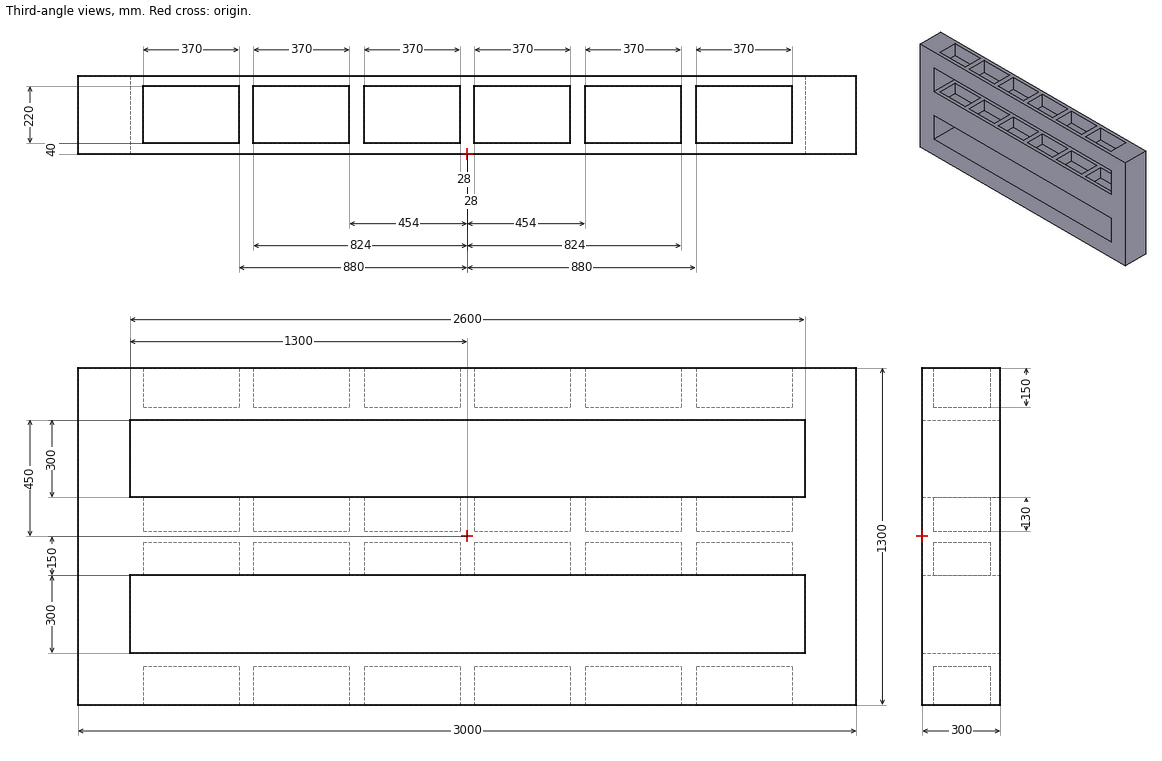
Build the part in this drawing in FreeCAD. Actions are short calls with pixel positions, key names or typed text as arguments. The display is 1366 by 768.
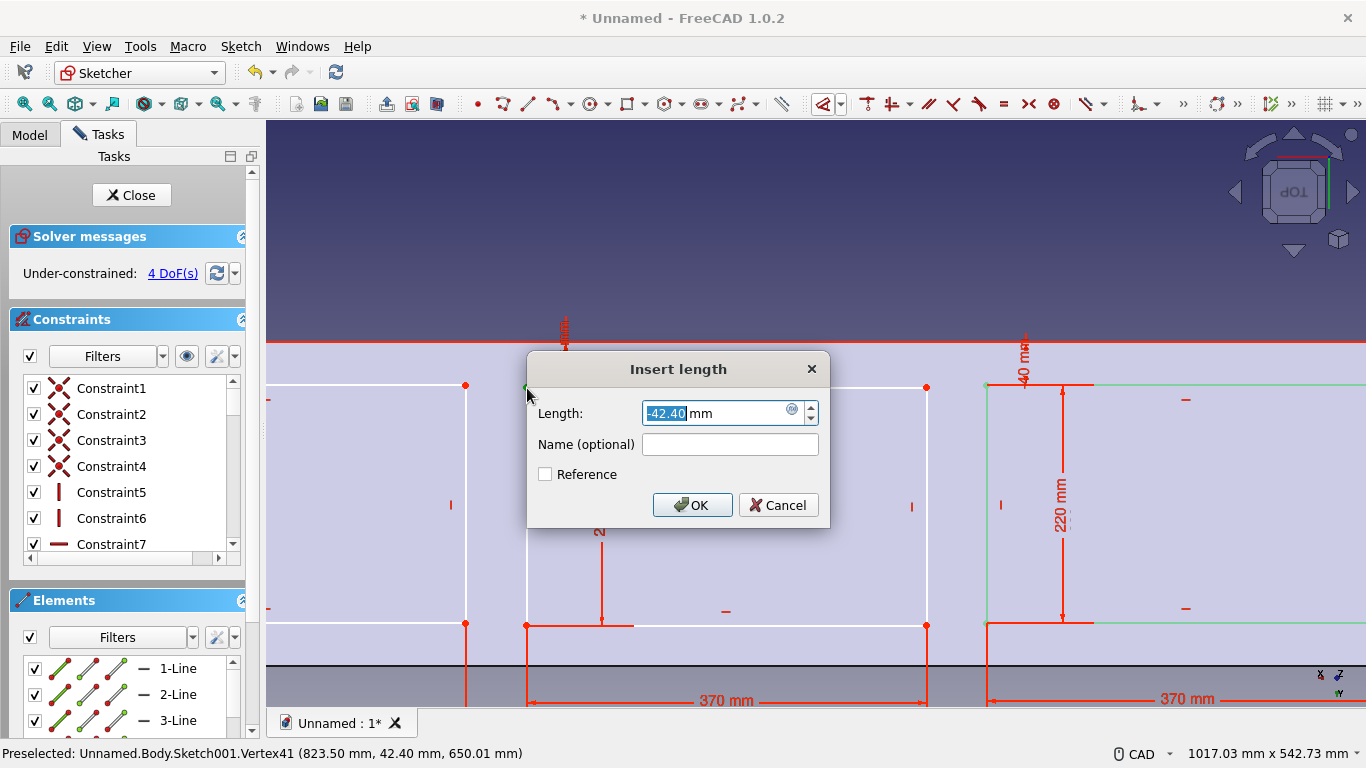
text(-40)
key(Return)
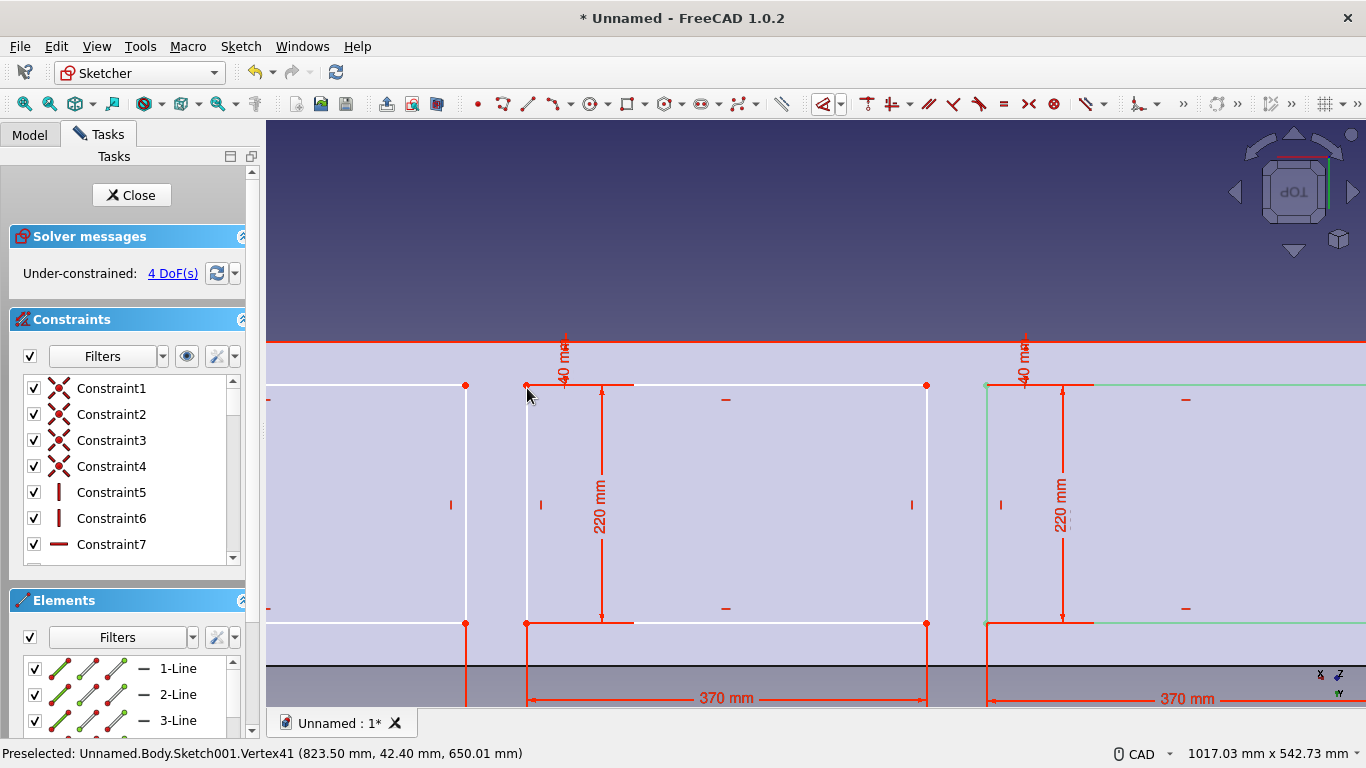
scroll(528, 391, down, 7)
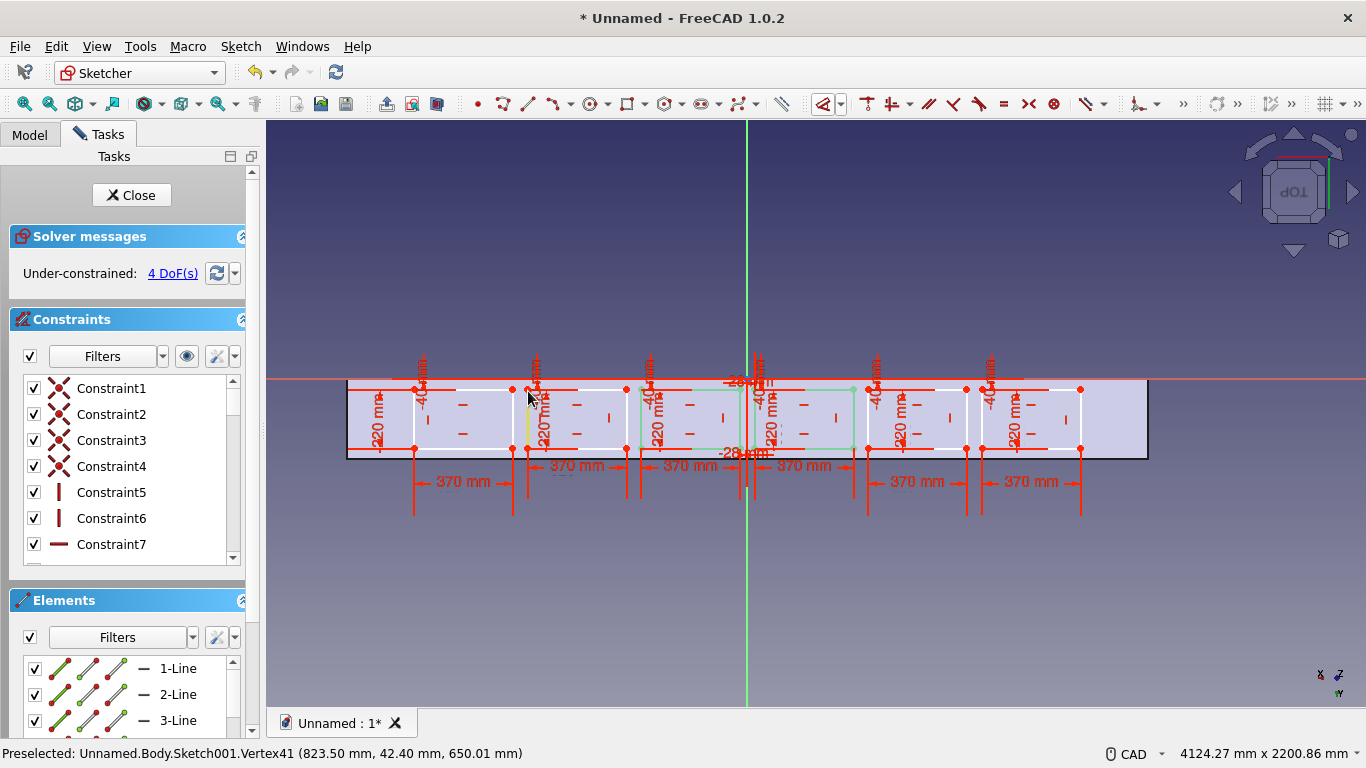
click(982, 390)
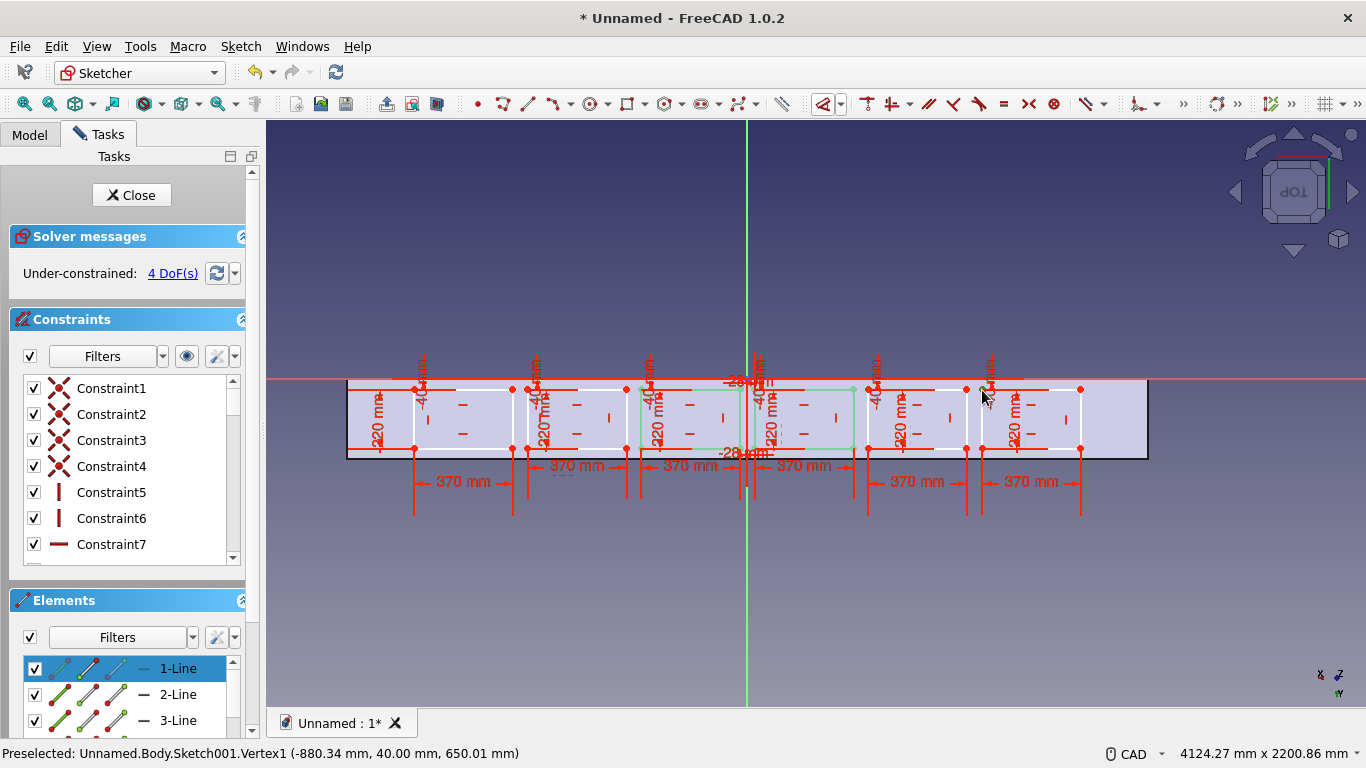
key(l)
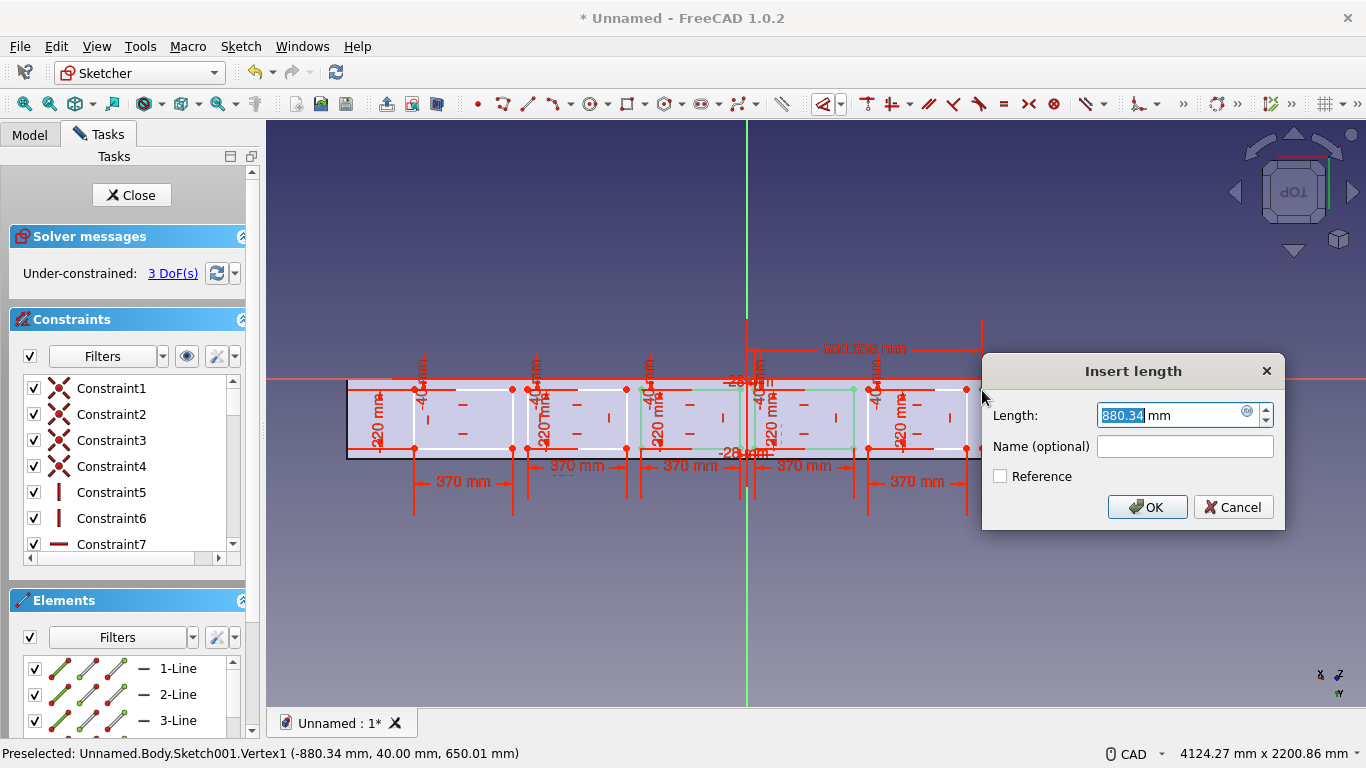
text(880)
key(Return)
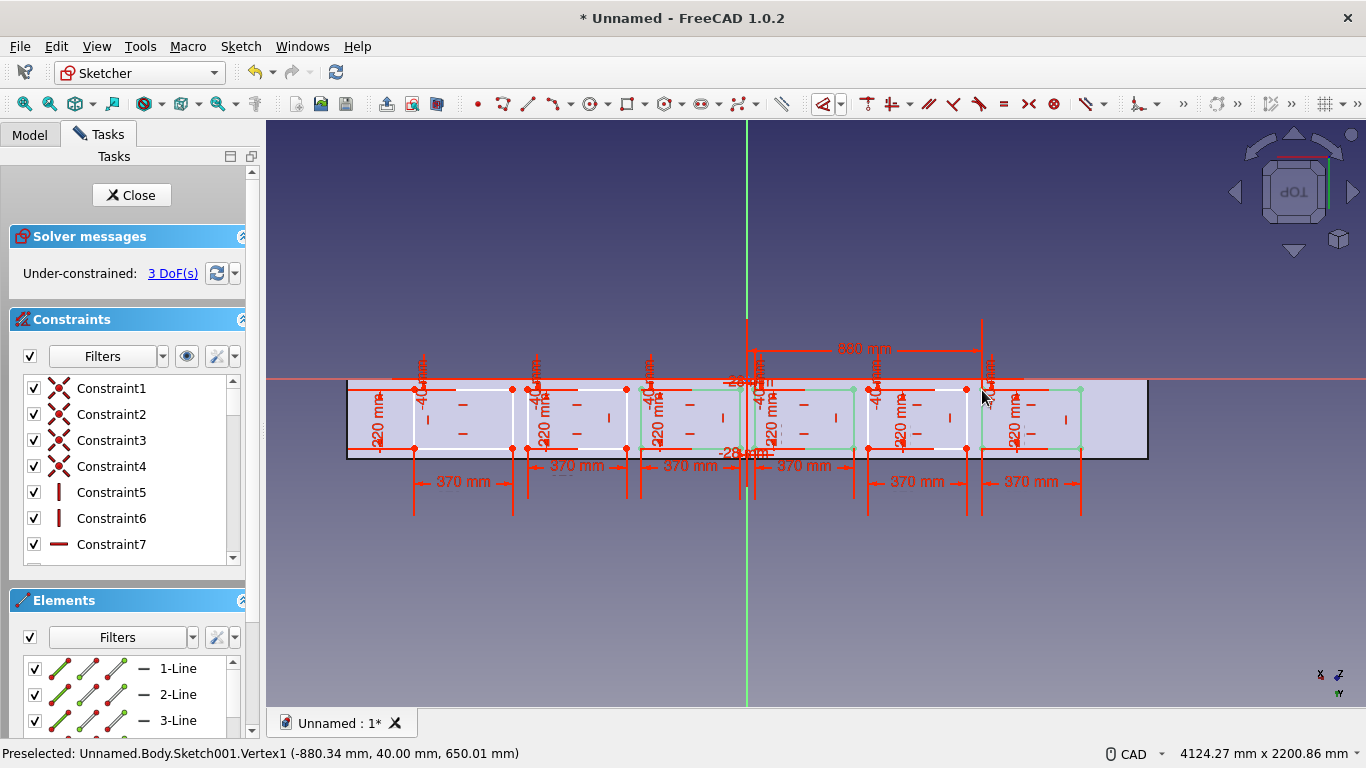
click(513, 449)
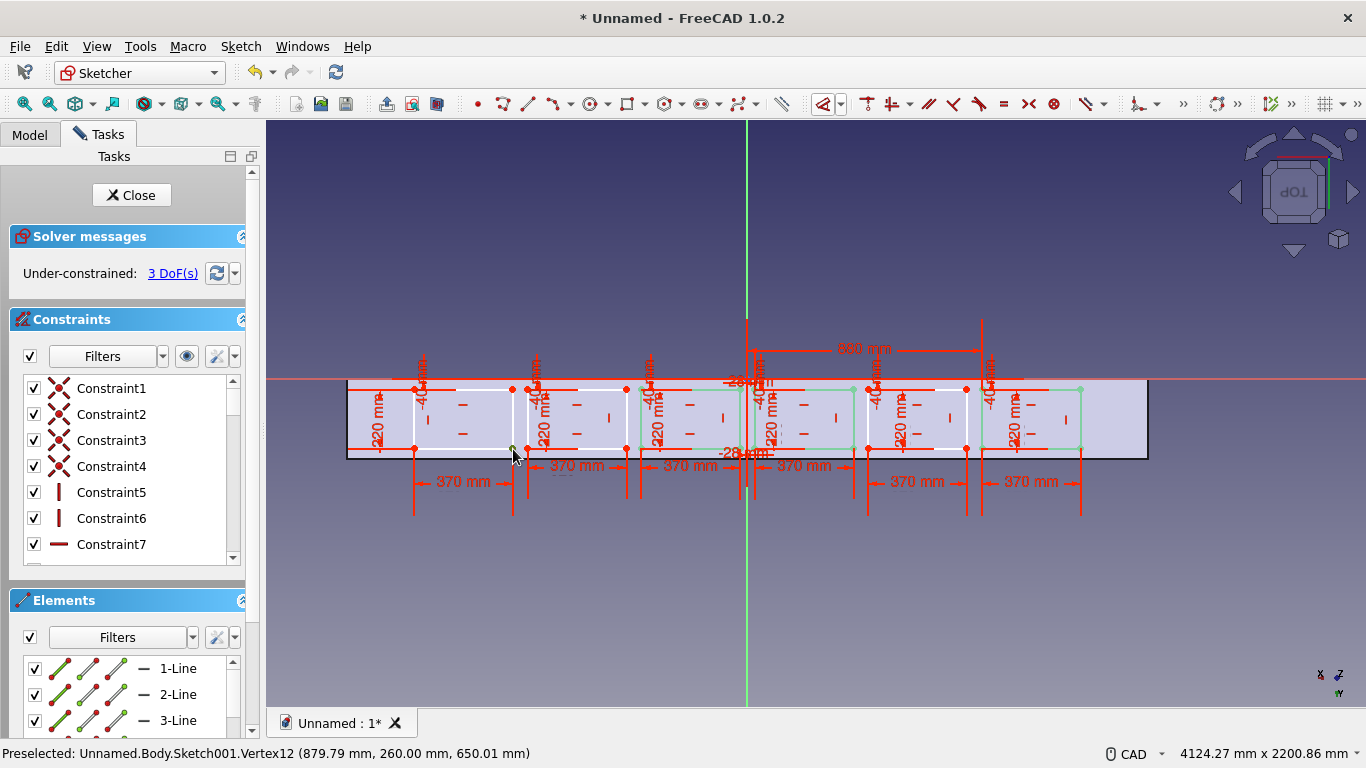
key(l)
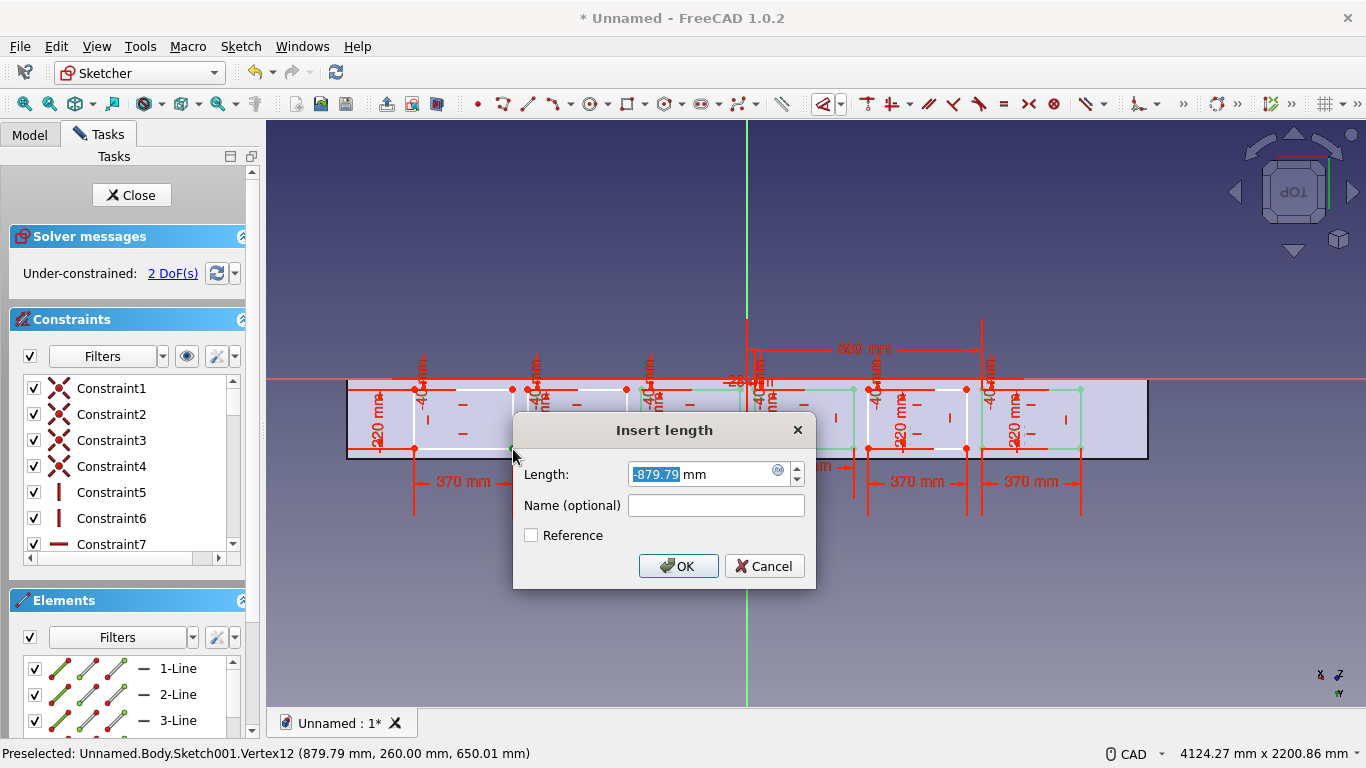
text(-880)
key(Return)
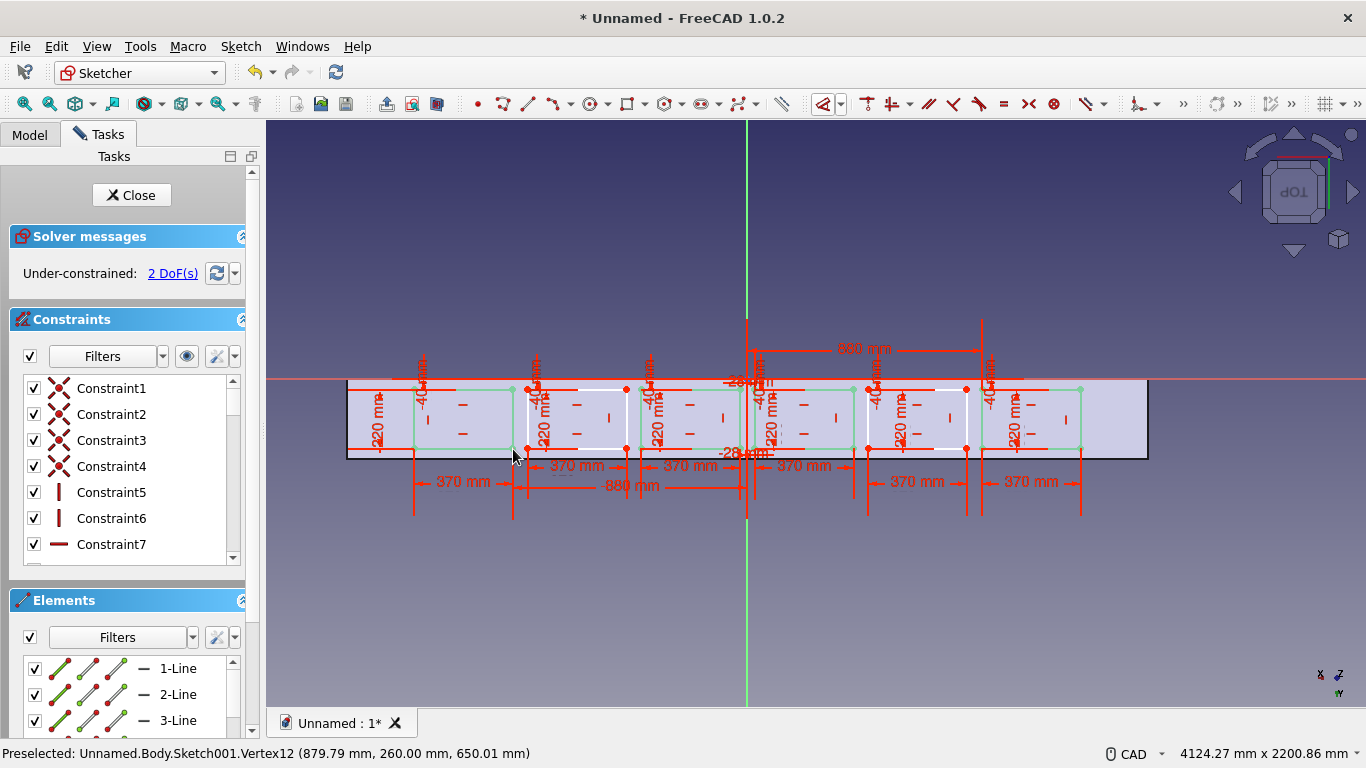
click(868, 390)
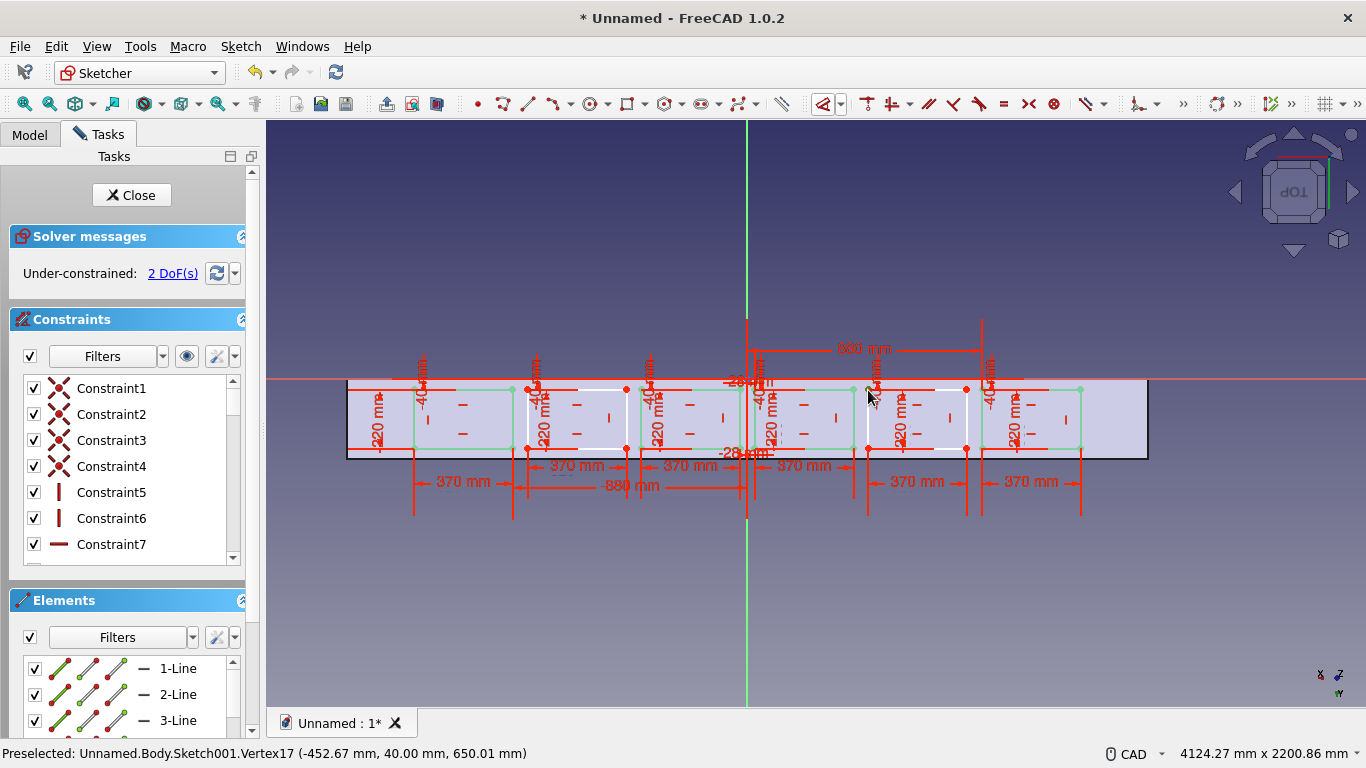
key(l)